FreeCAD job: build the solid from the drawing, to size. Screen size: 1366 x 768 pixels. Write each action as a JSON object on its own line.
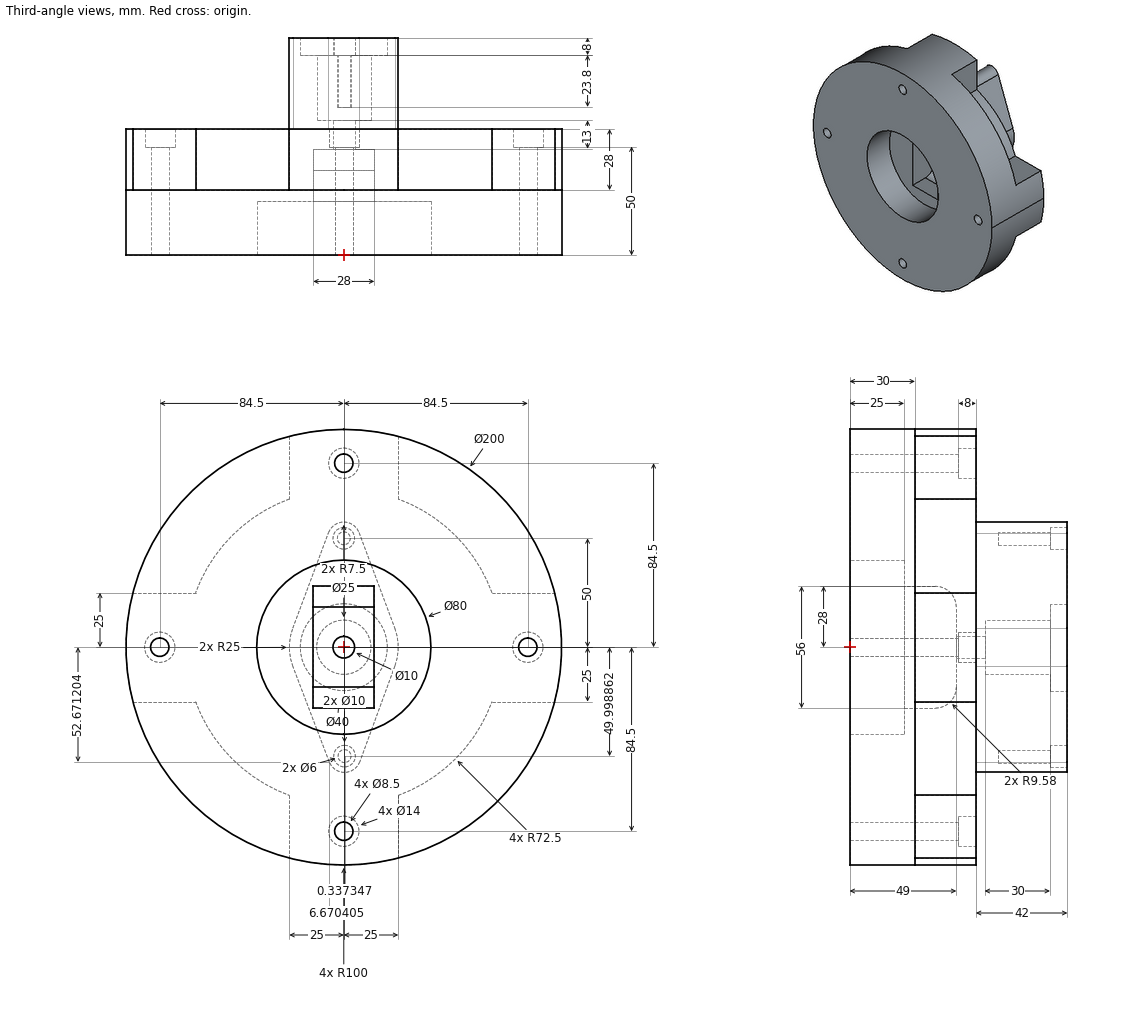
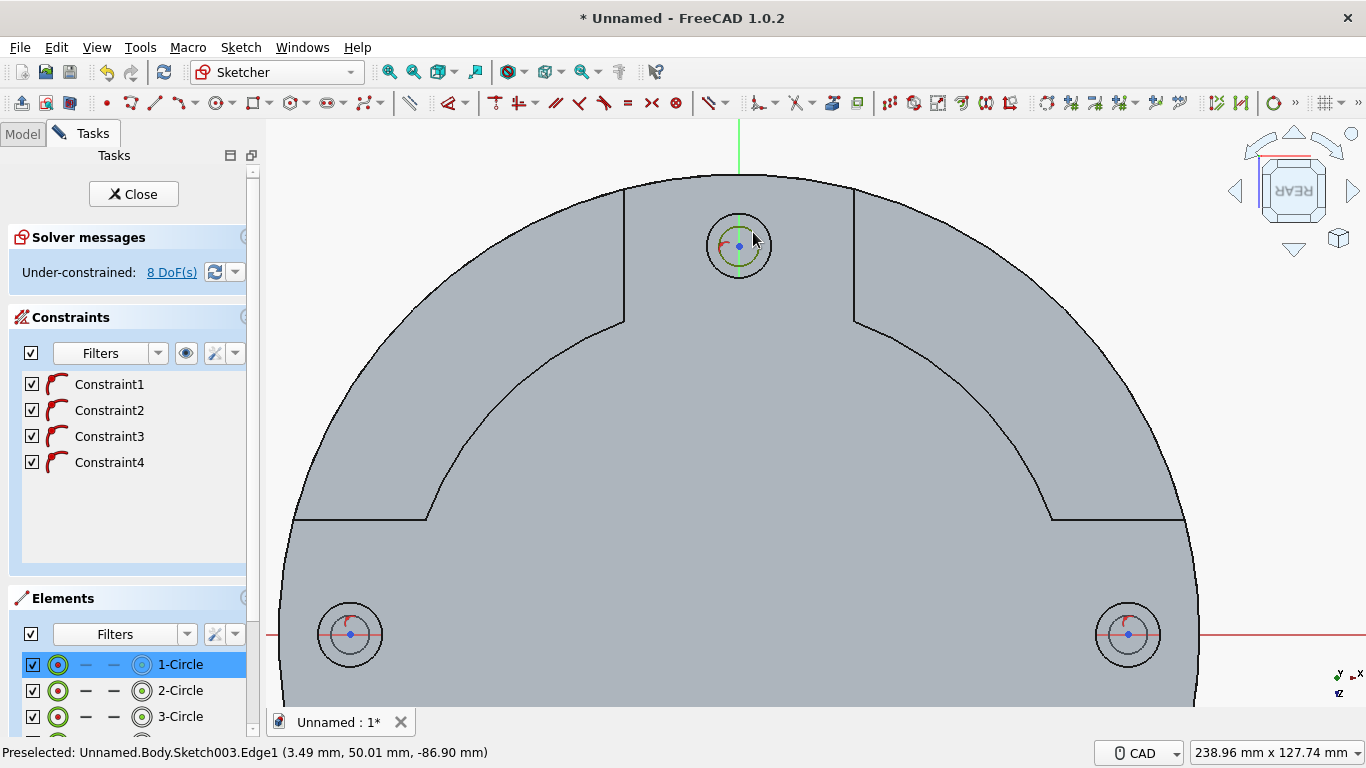
{"action": "left_click", "coordinate": [1142, 621]}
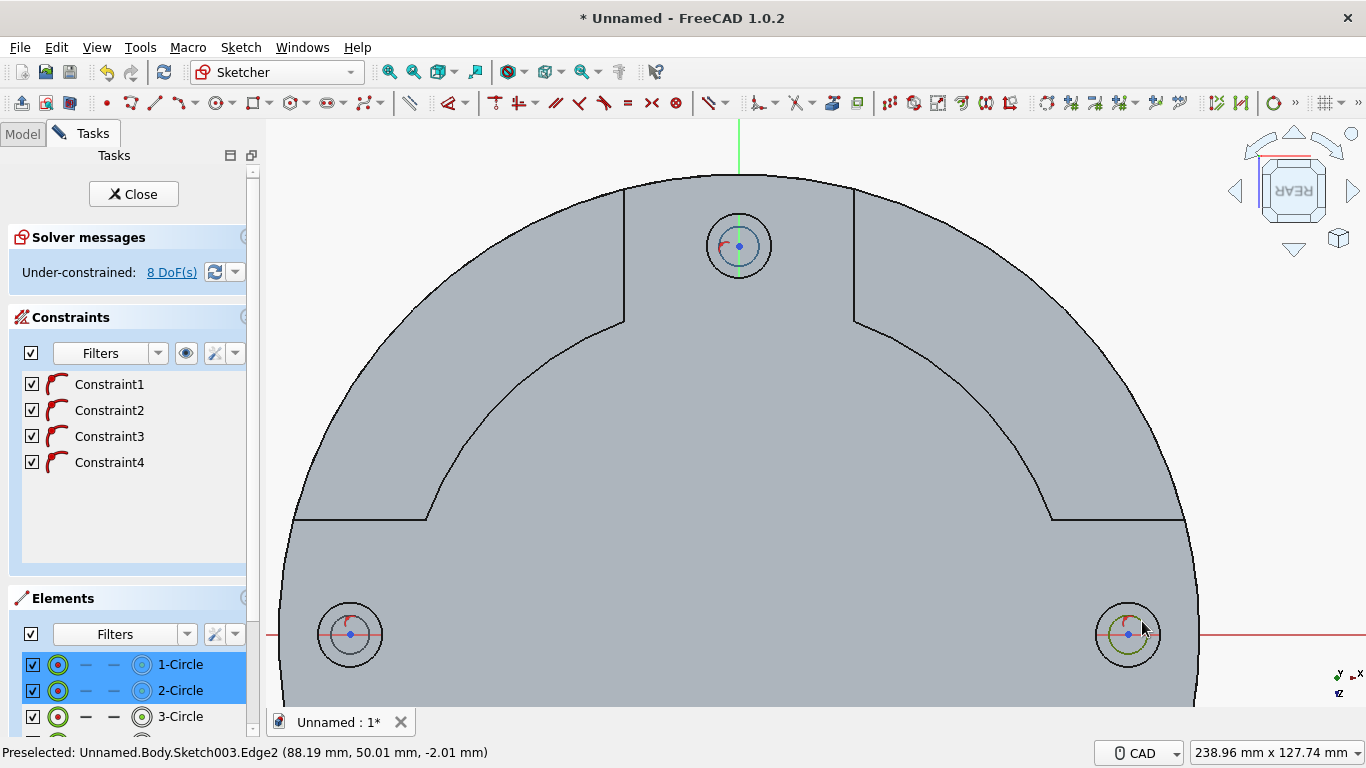
{"action": "scroll", "coordinate": [754, 232], "scroll_direction": "down", "scroll_amount": 4}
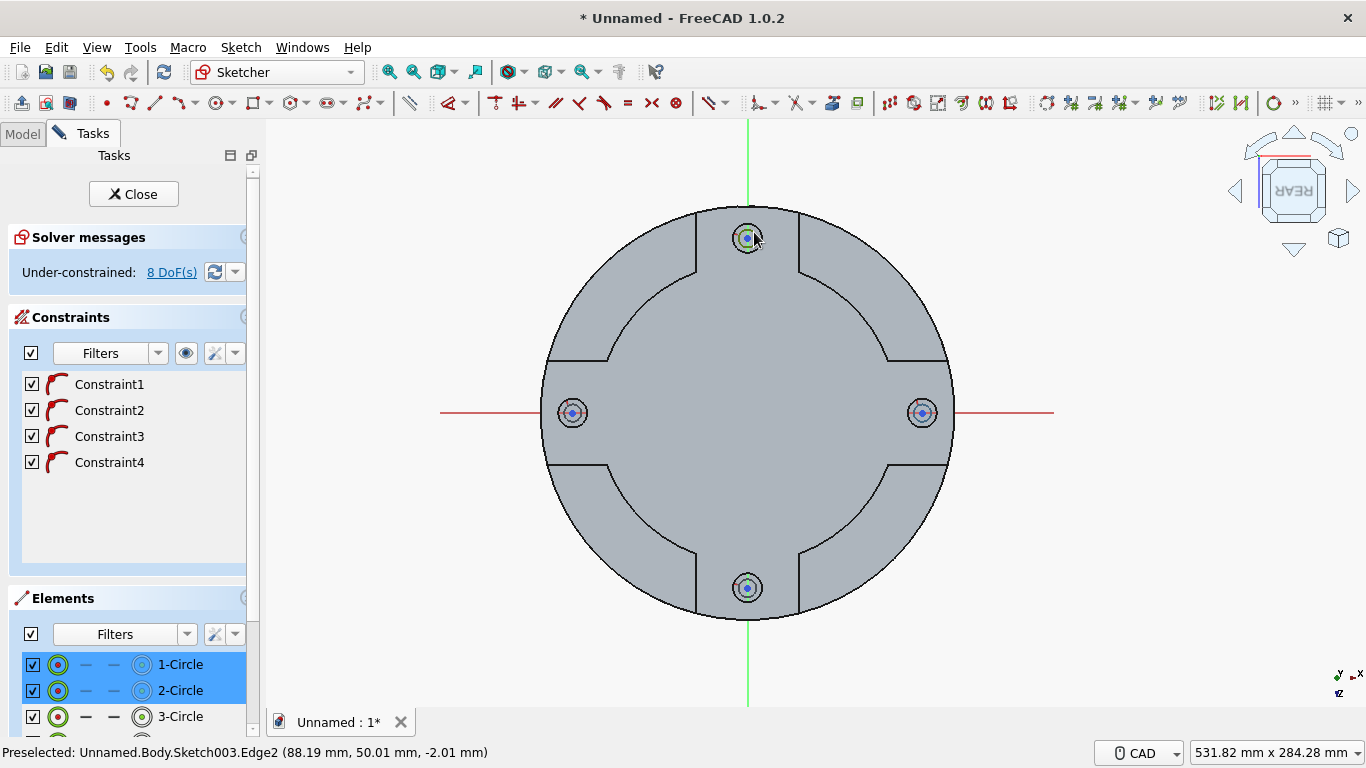
{"action": "scroll", "coordinate": [754, 582], "scroll_direction": "up", "scroll_amount": 4}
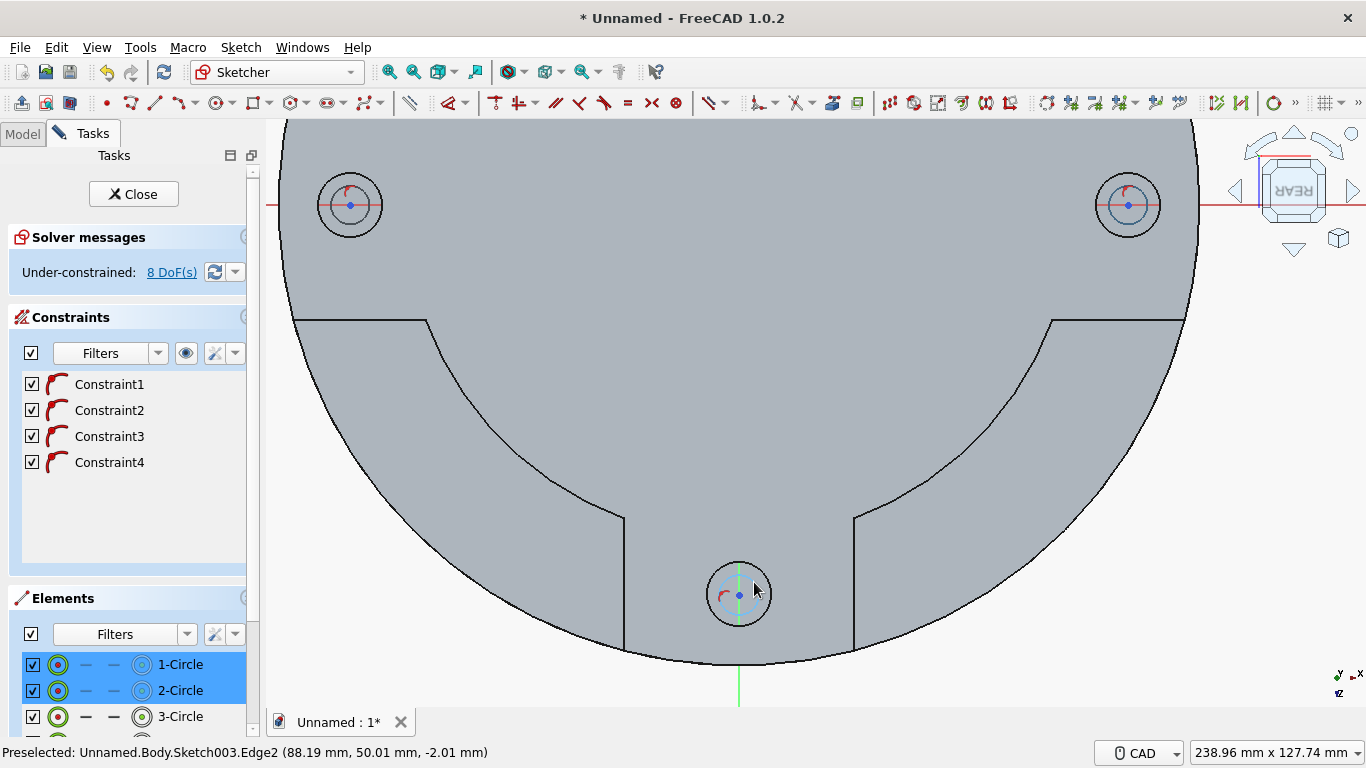
{"action": "left_click", "coordinate": [753, 581]}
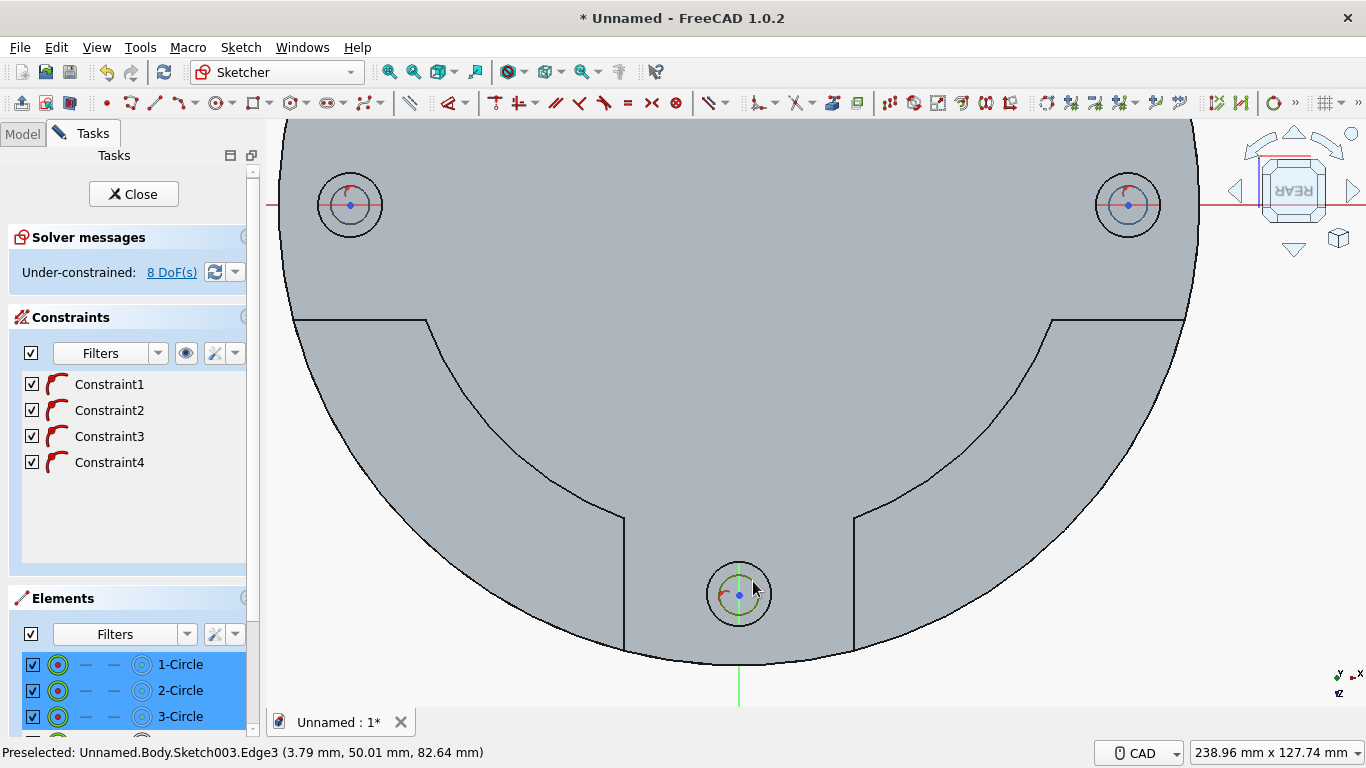
{"action": "left_click", "coordinate": [364, 191]}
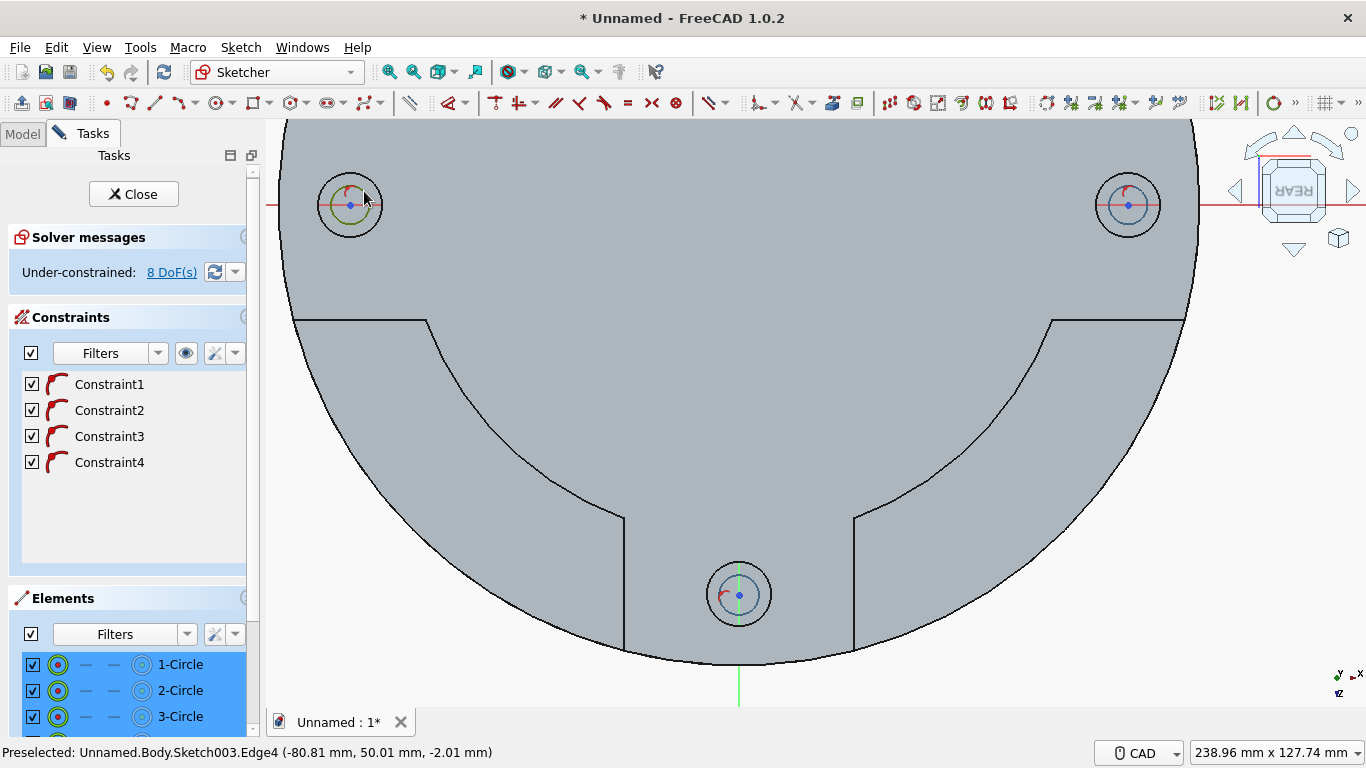
{"action": "key", "text": "e"}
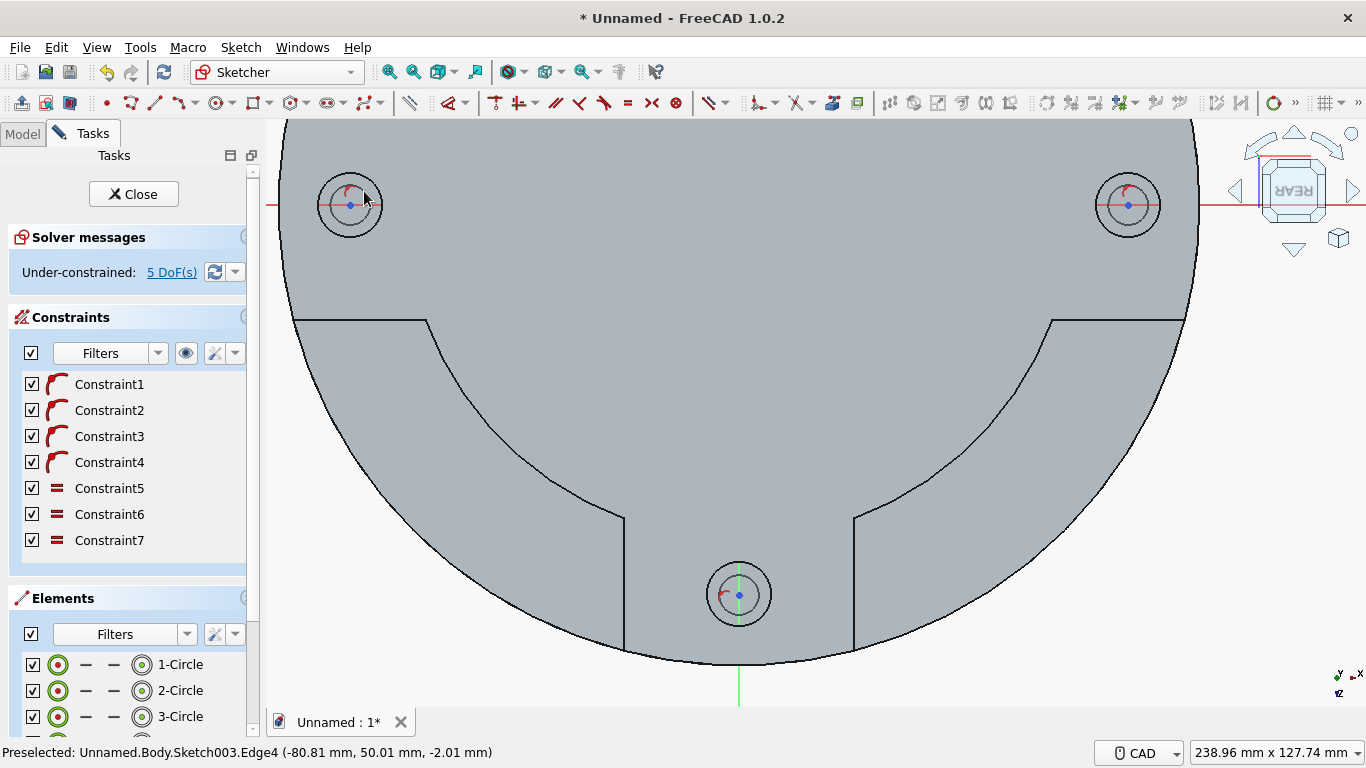
{"action": "key", "text": "d"}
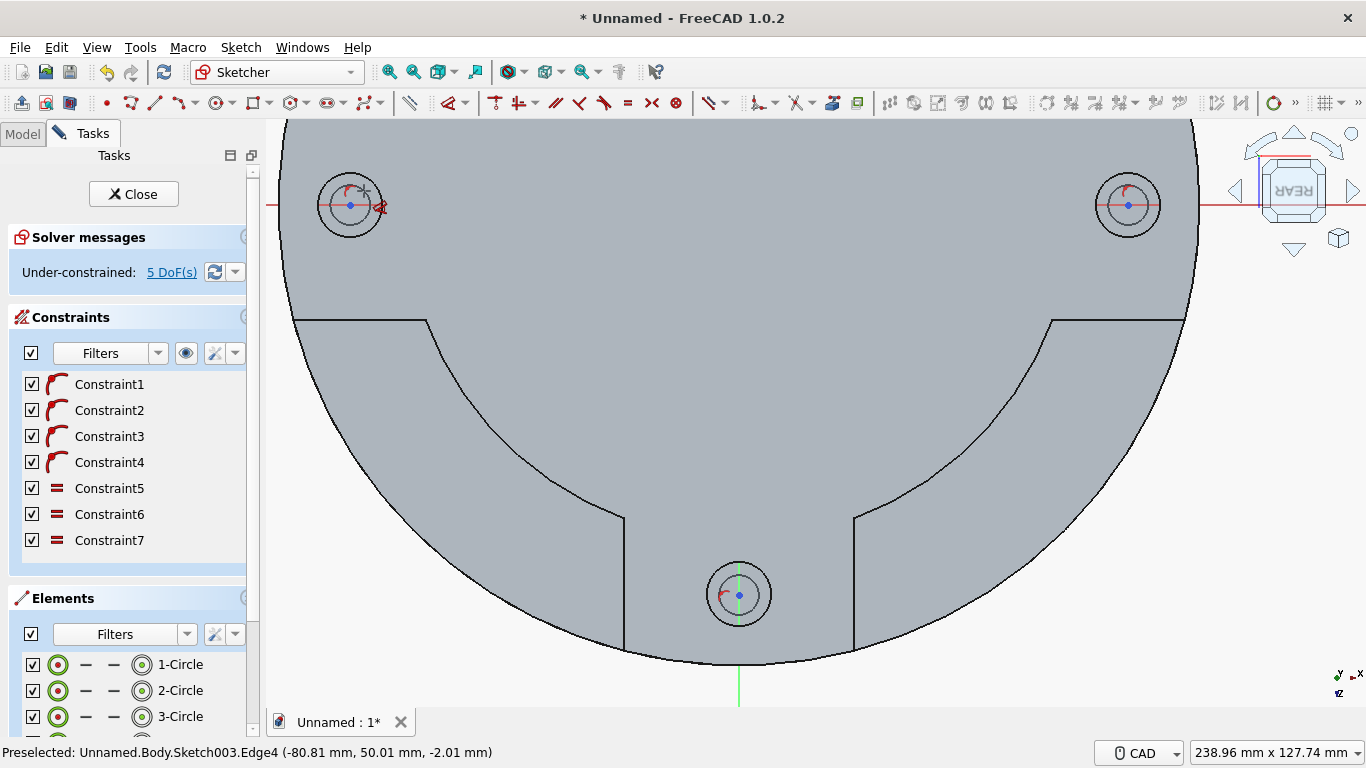
{"action": "scroll", "coordinate": [754, 583], "scroll_direction": "down", "scroll_amount": 4}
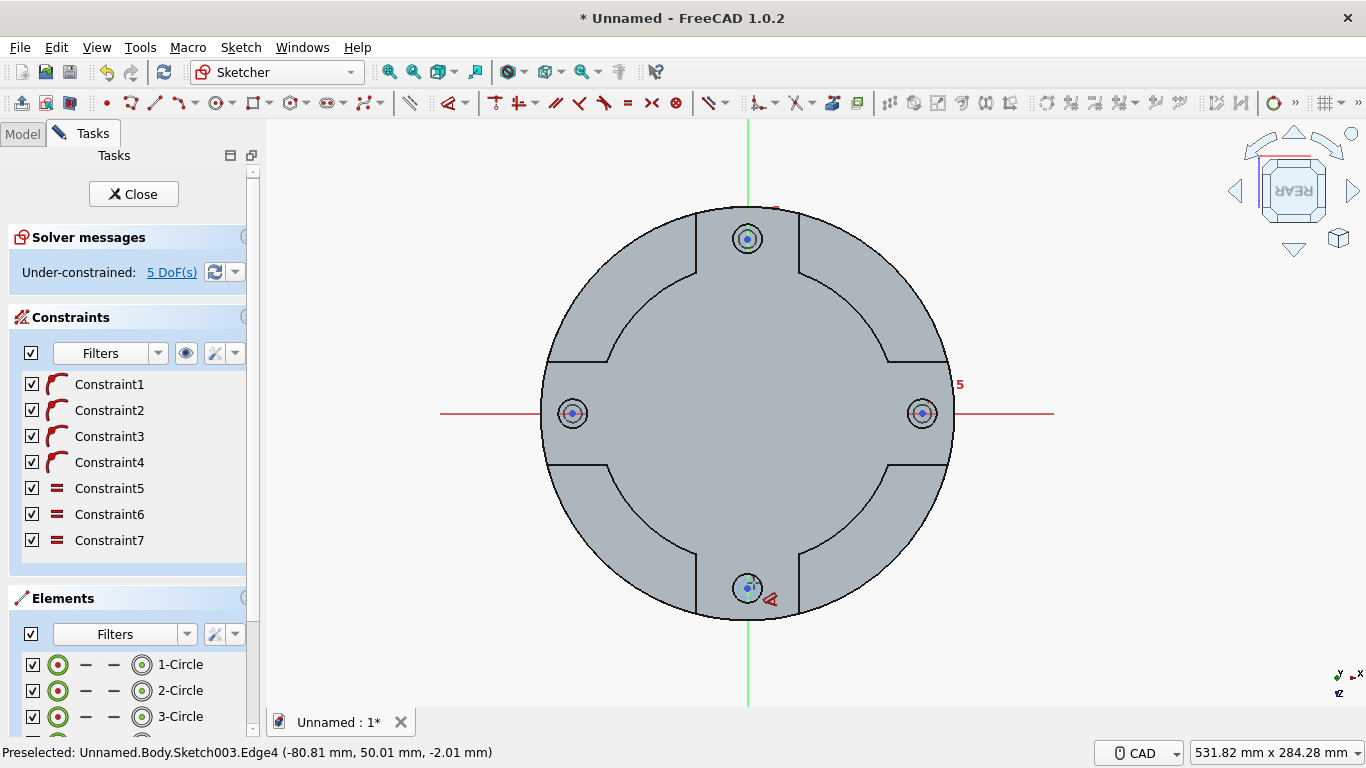
{"action": "scroll", "coordinate": [754, 233], "scroll_direction": "up", "scroll_amount": 5}